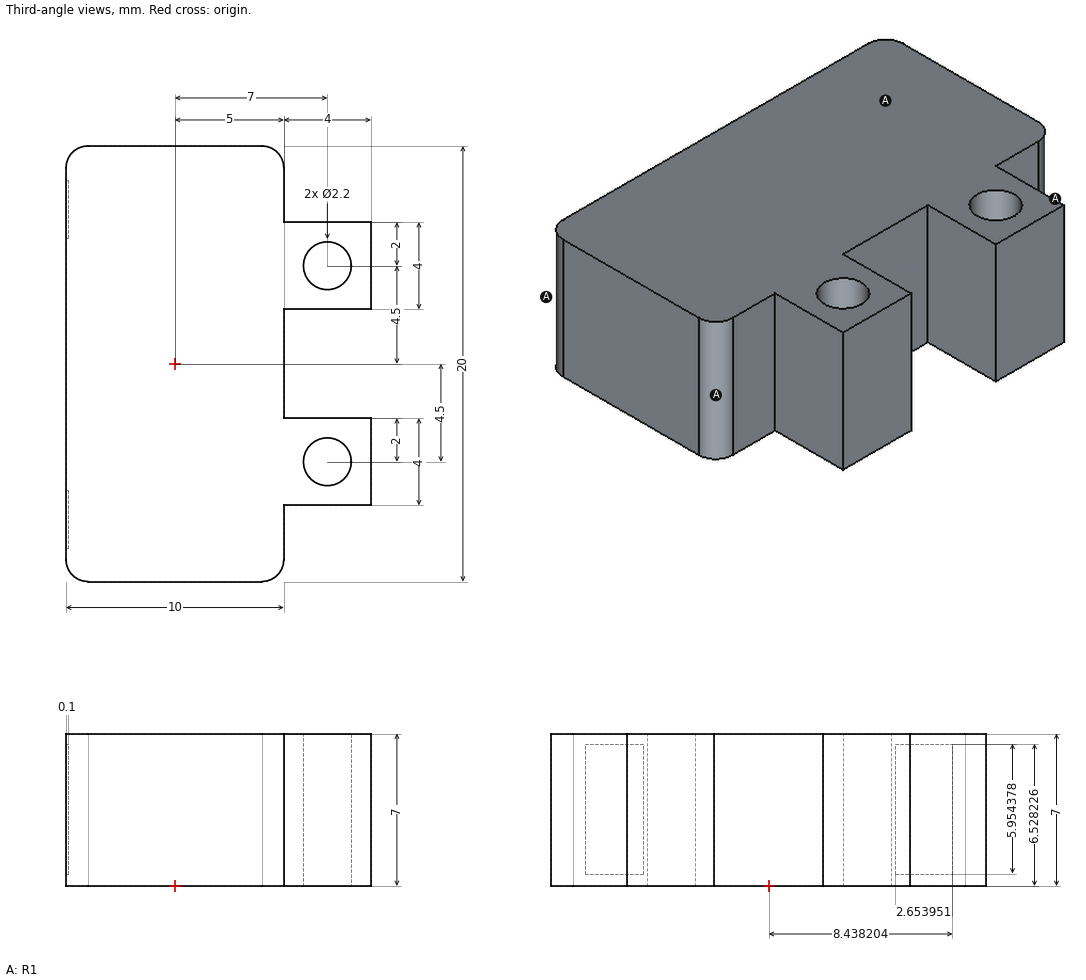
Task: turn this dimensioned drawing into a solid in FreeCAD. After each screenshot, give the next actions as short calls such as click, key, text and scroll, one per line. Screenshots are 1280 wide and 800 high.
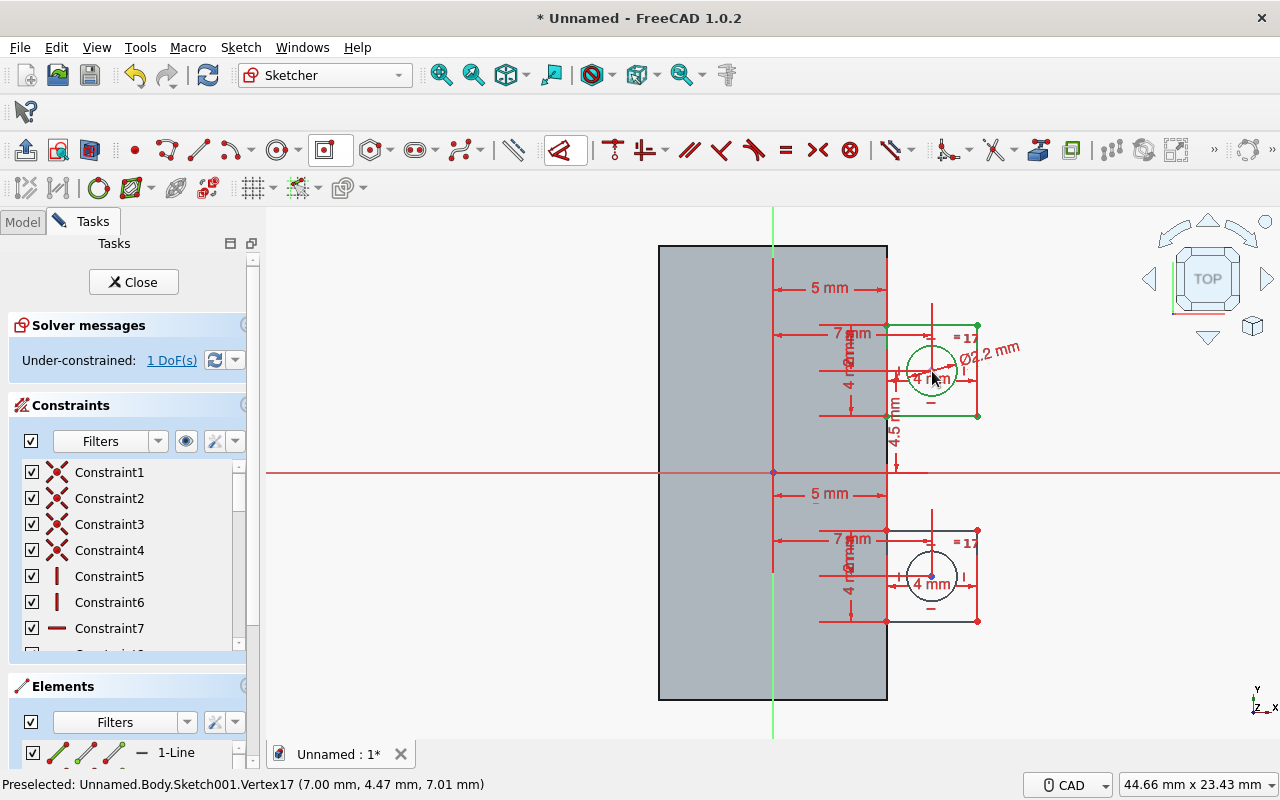
click(932, 576)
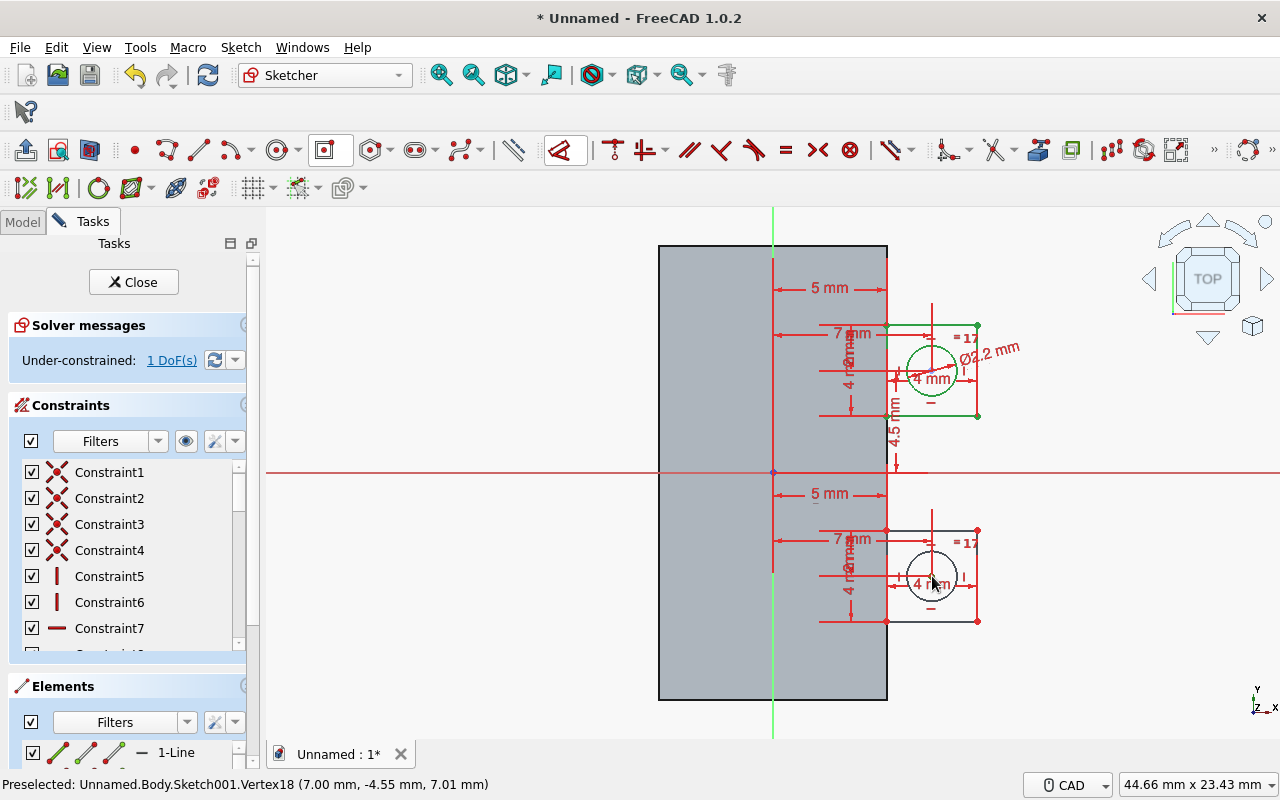
key(i)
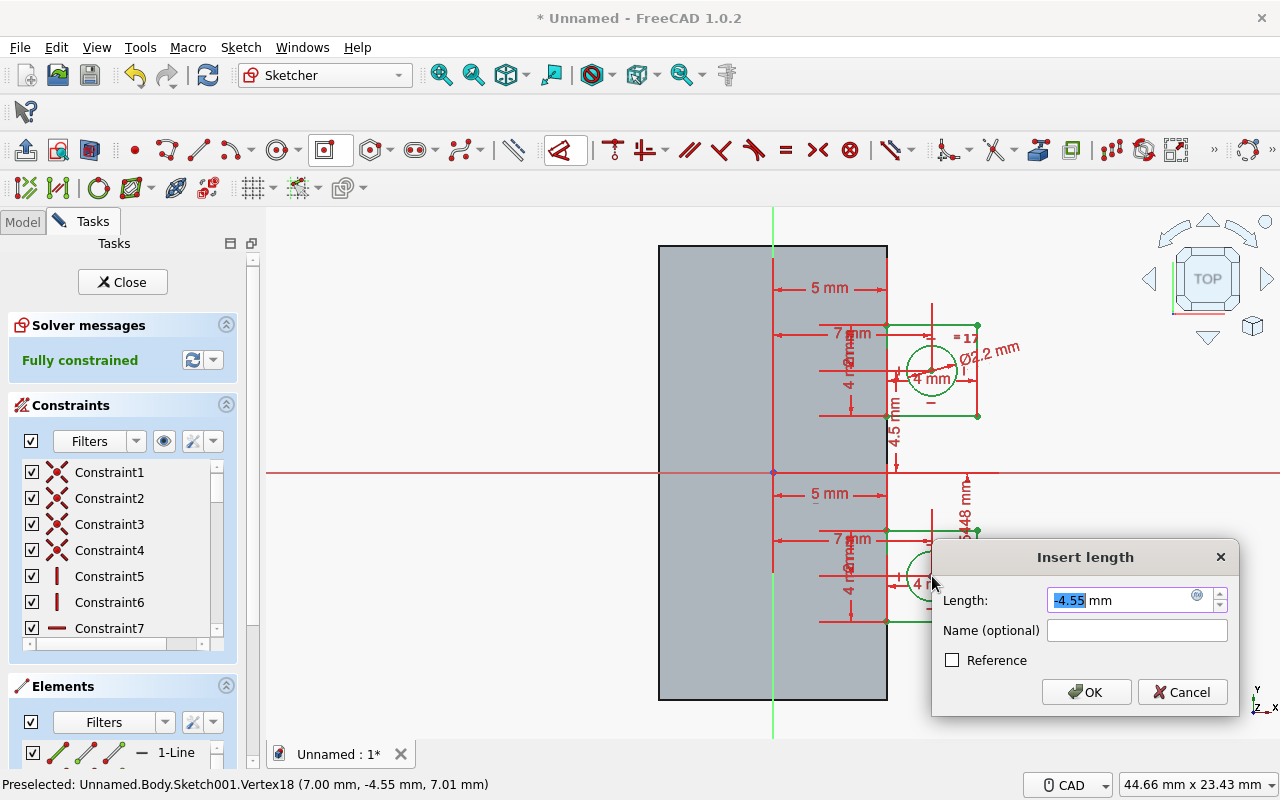
text(-4.5)
key(Return)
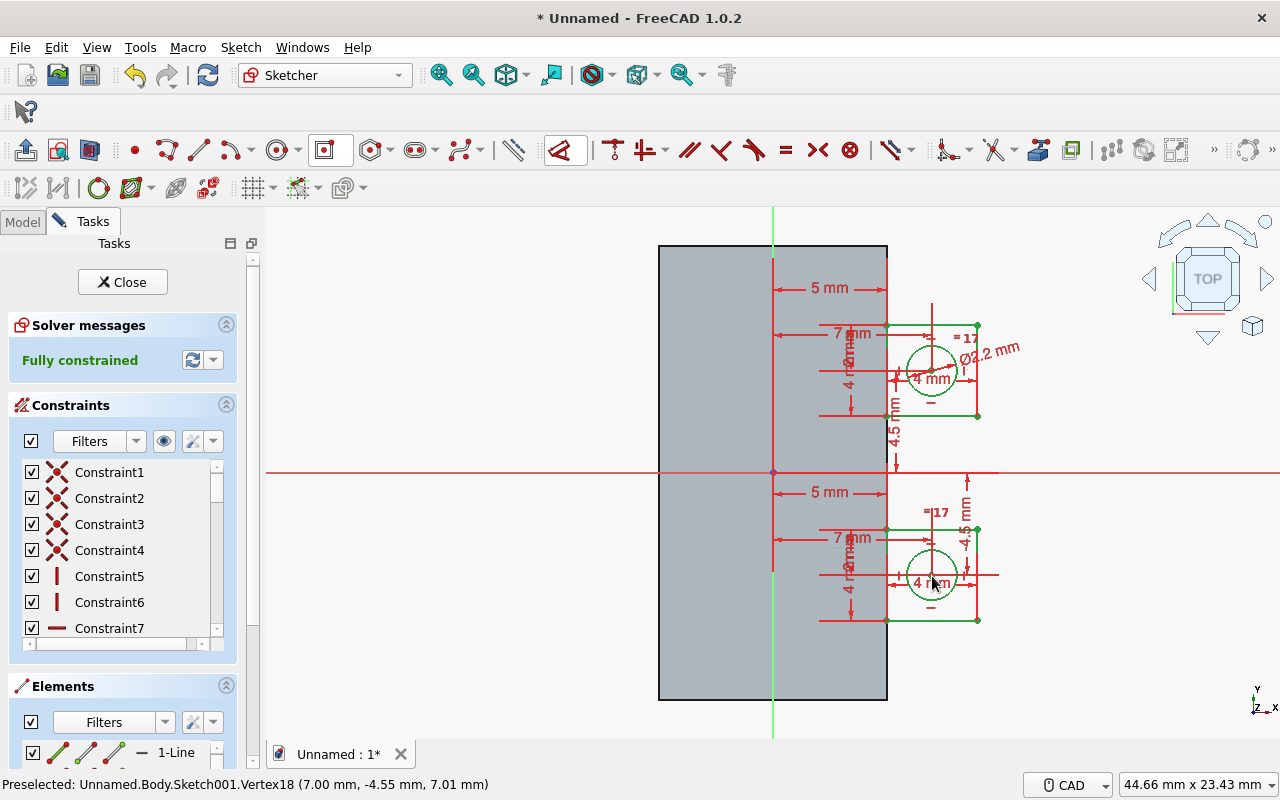
click(123, 282)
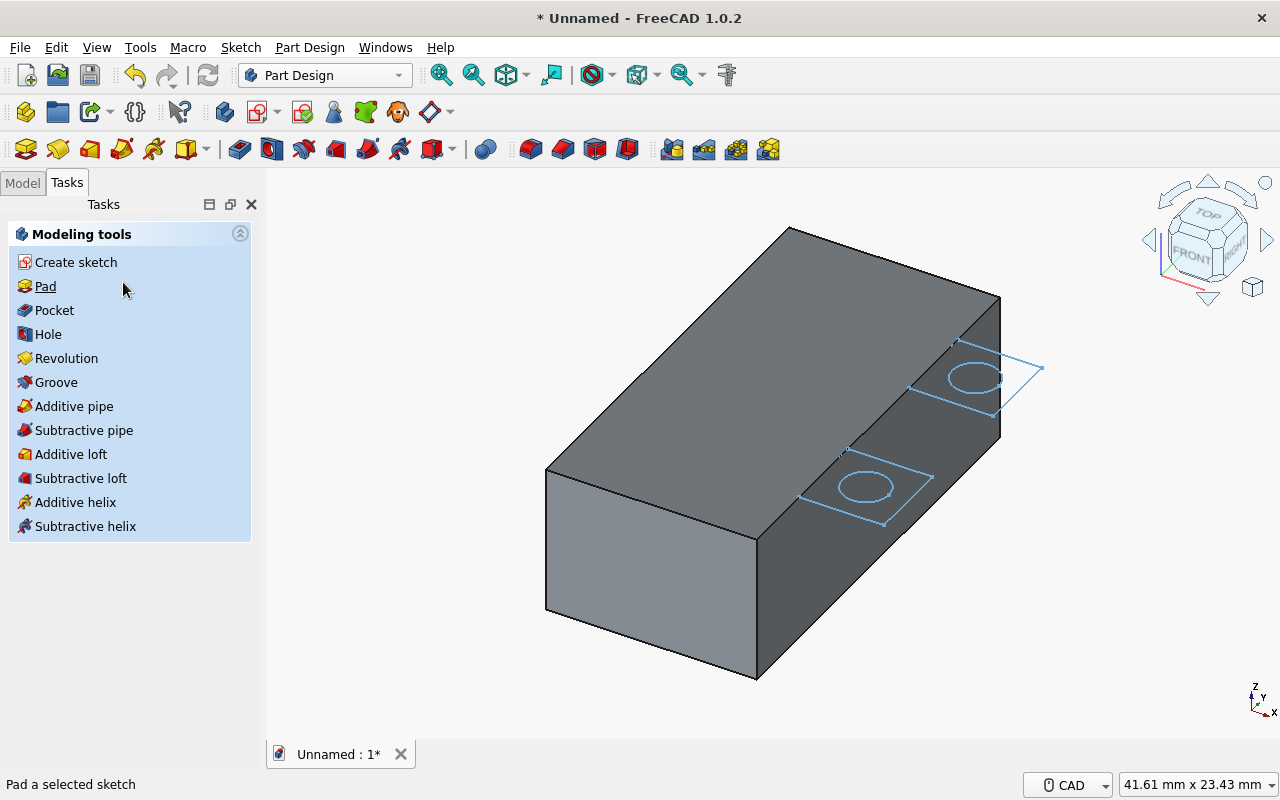
click(26, 150)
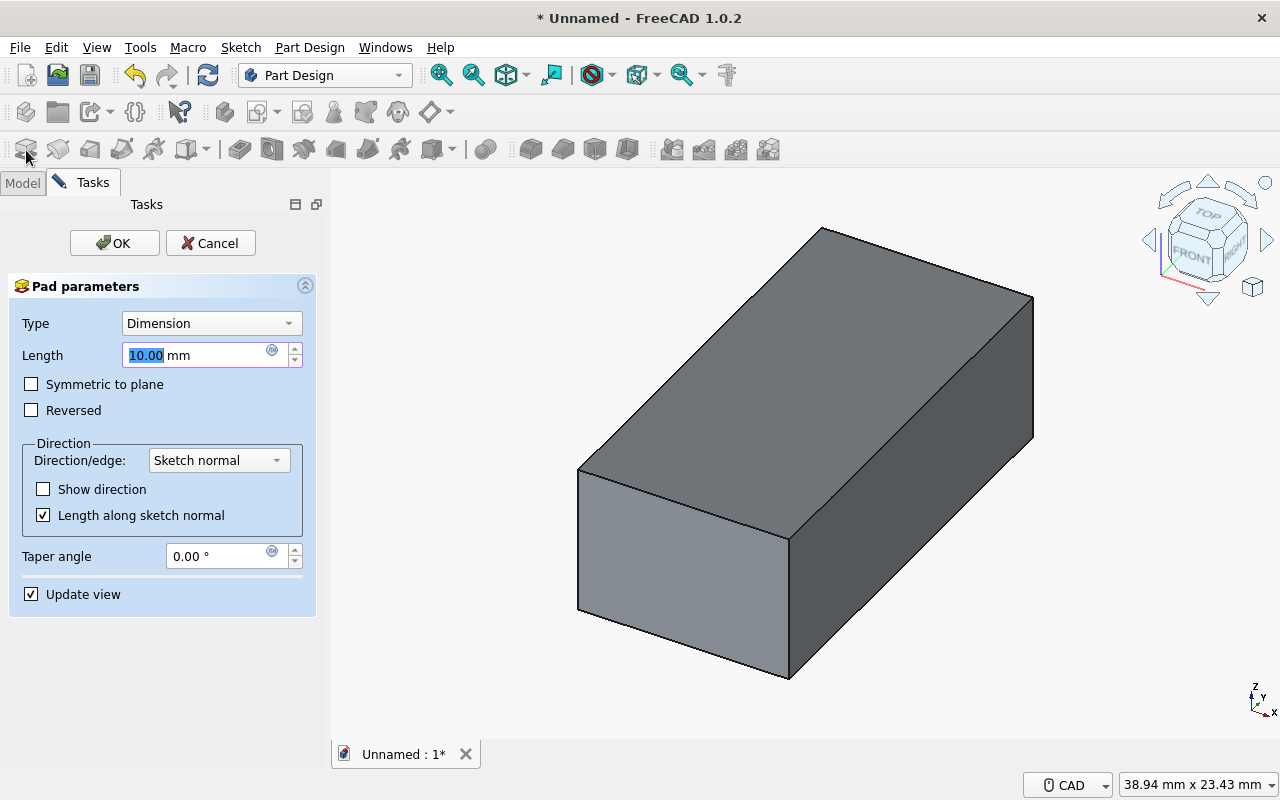
text(7)
key(Tab)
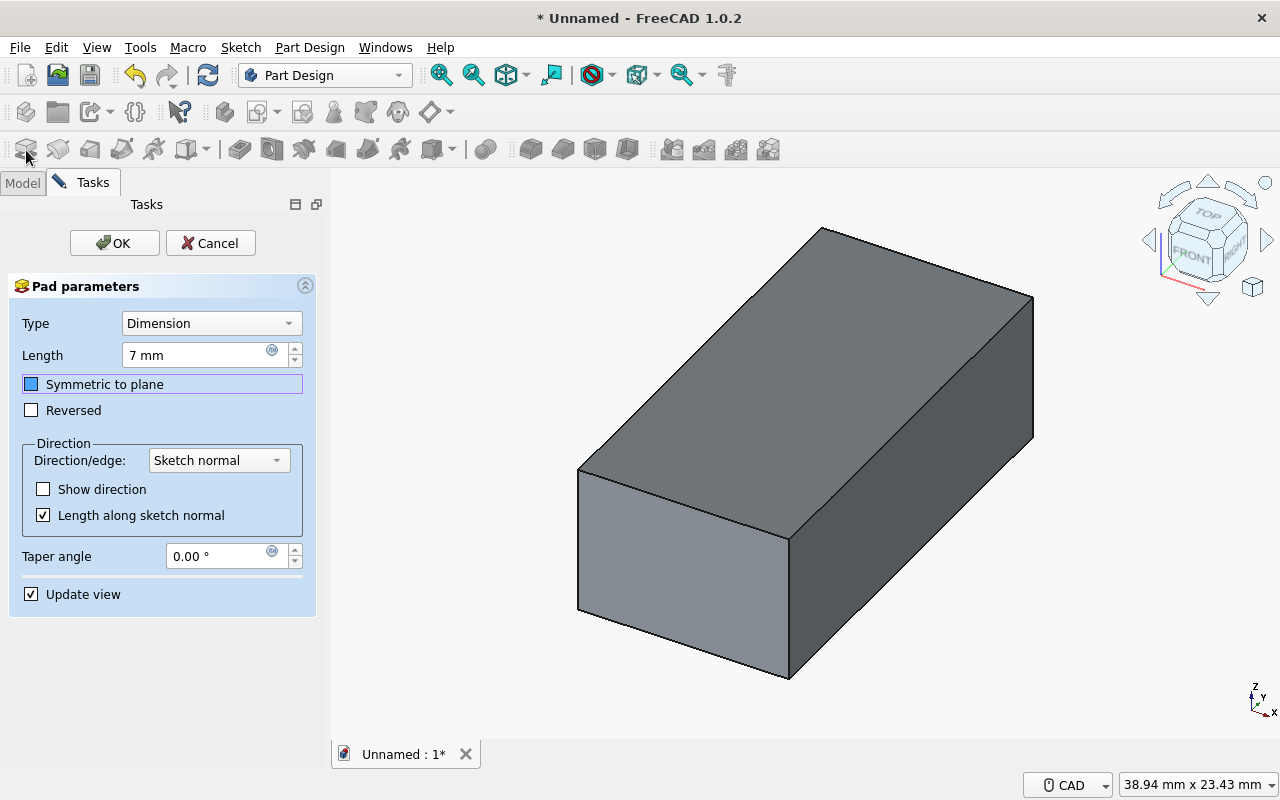
click(30, 410)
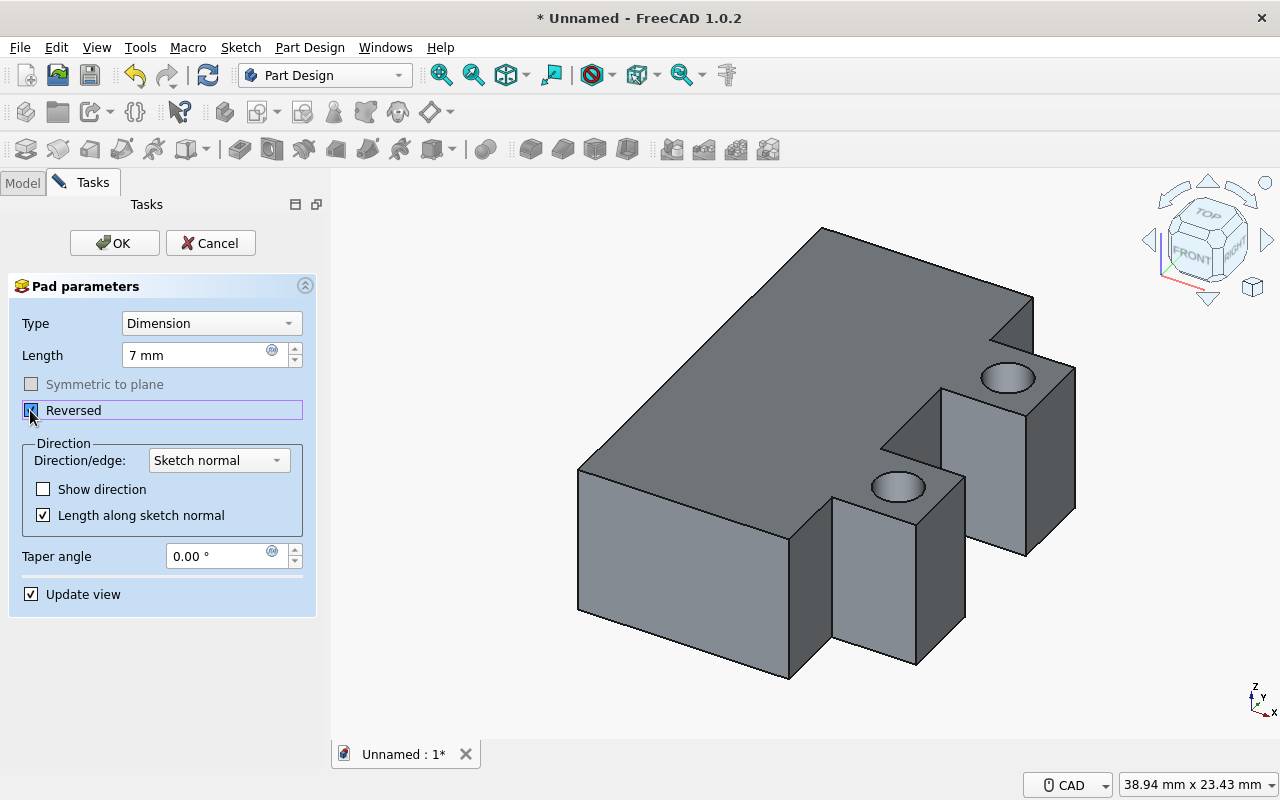
click(115, 243)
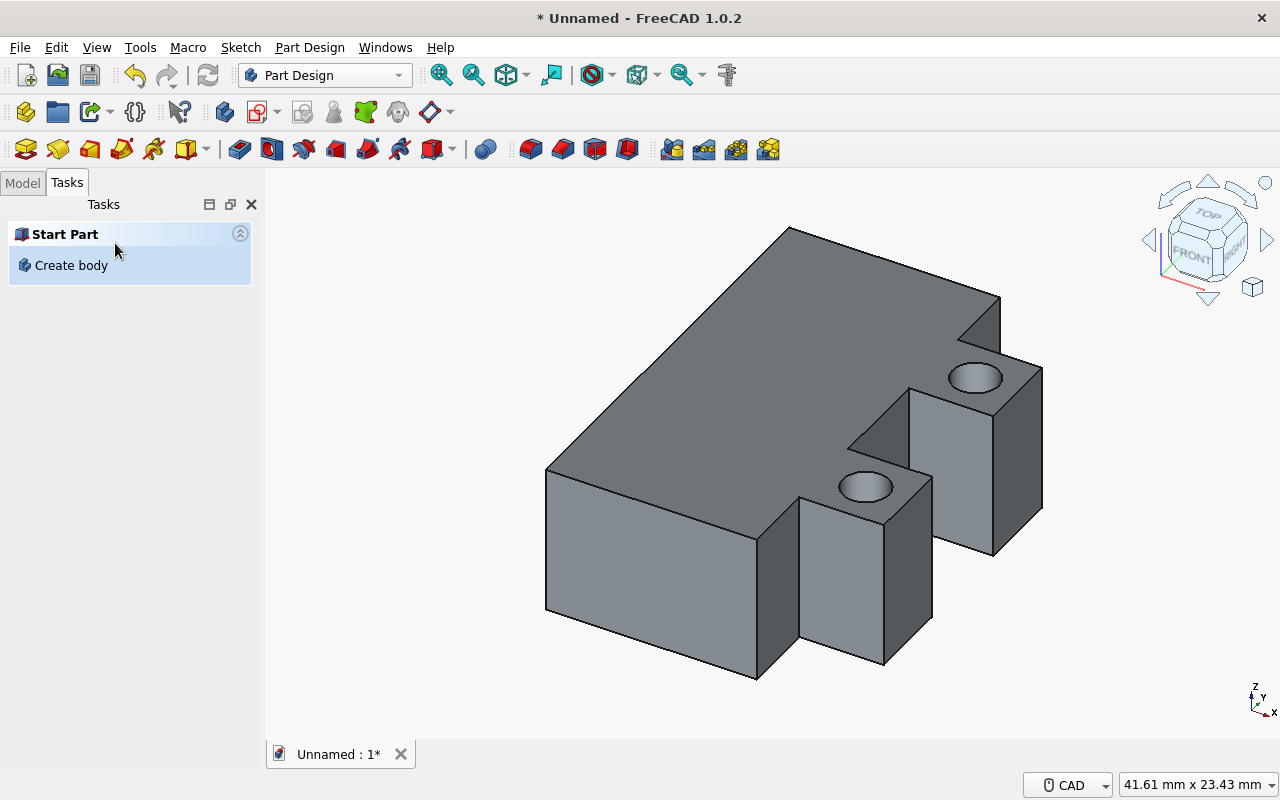
click(757, 608)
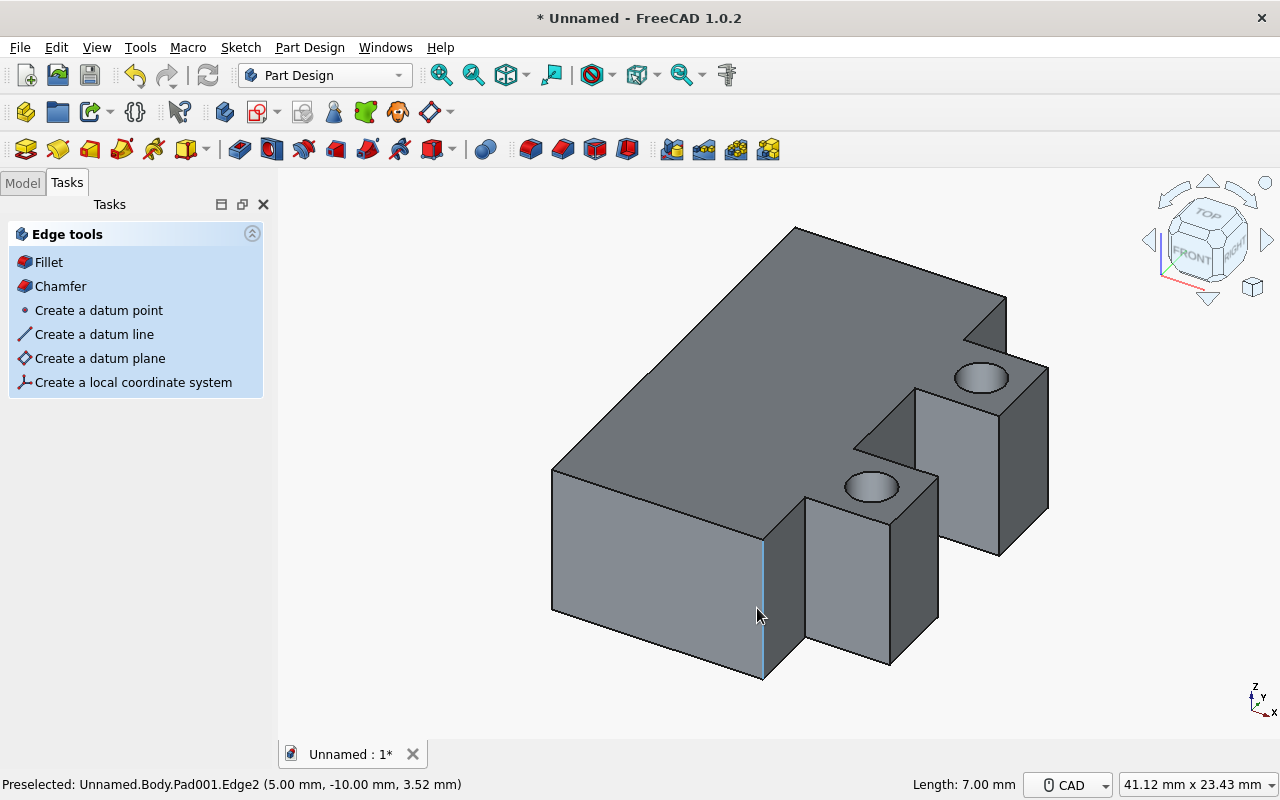
key(0)